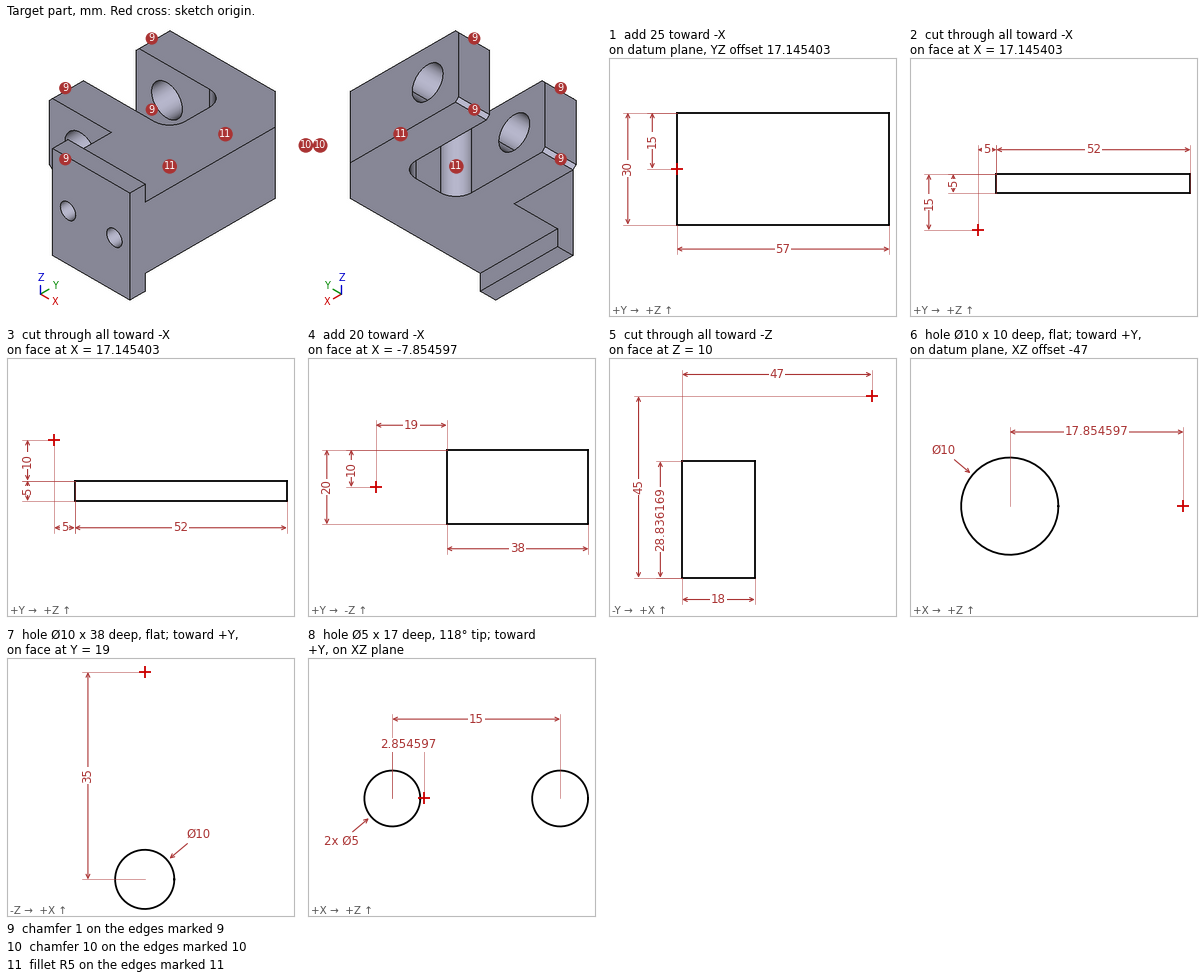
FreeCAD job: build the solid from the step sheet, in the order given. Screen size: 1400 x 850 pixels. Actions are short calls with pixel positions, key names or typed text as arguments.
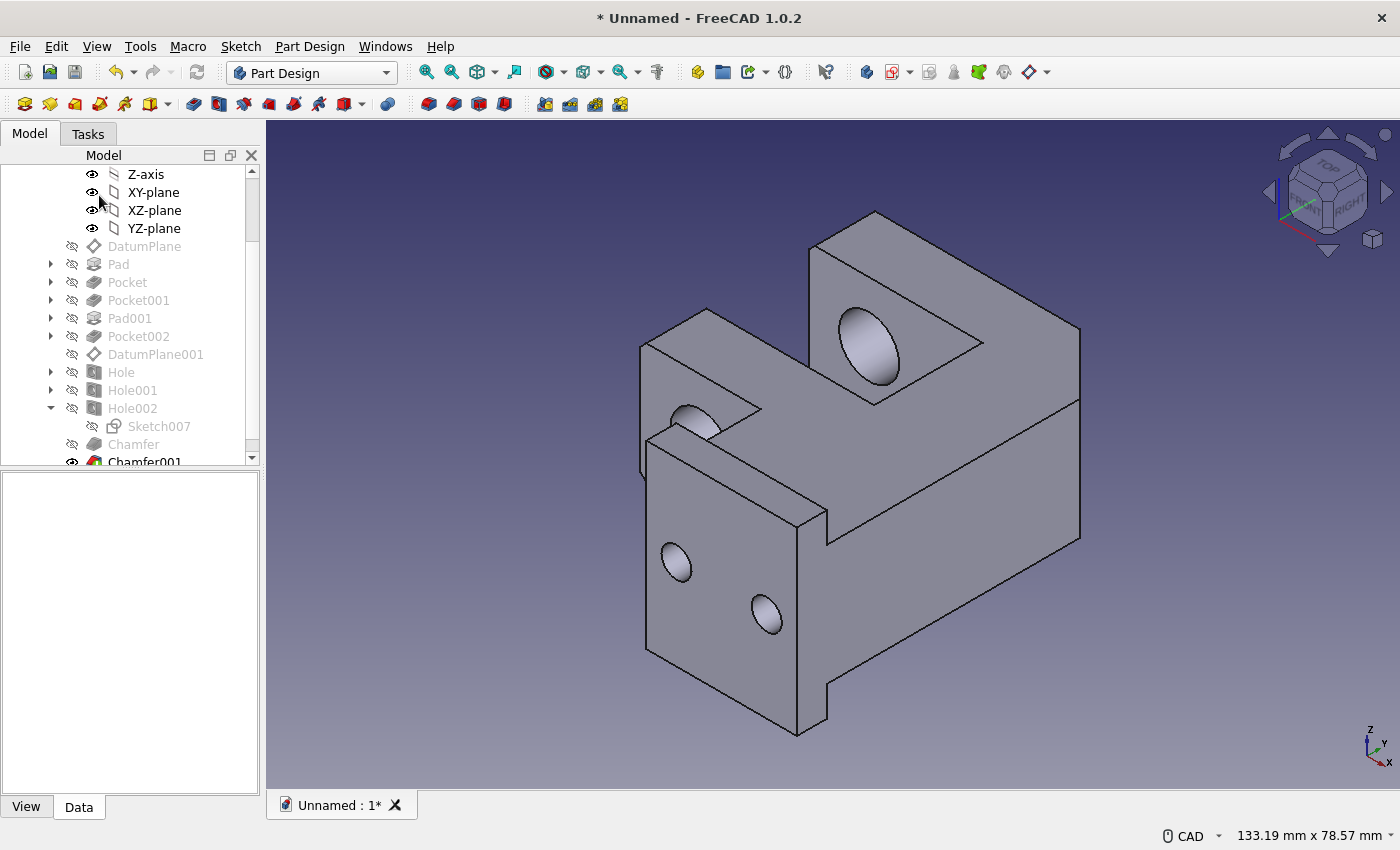
key(2)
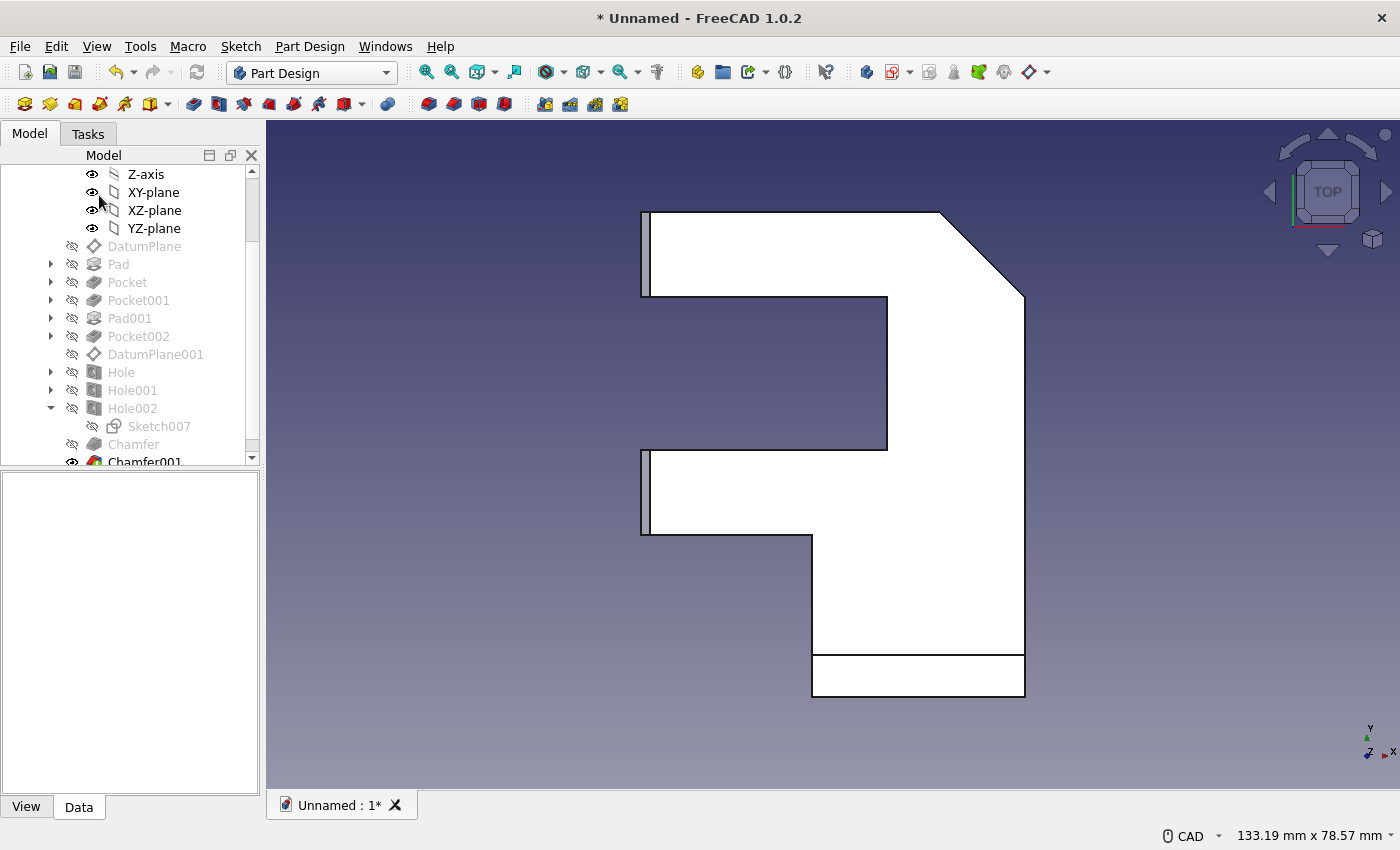
key(1)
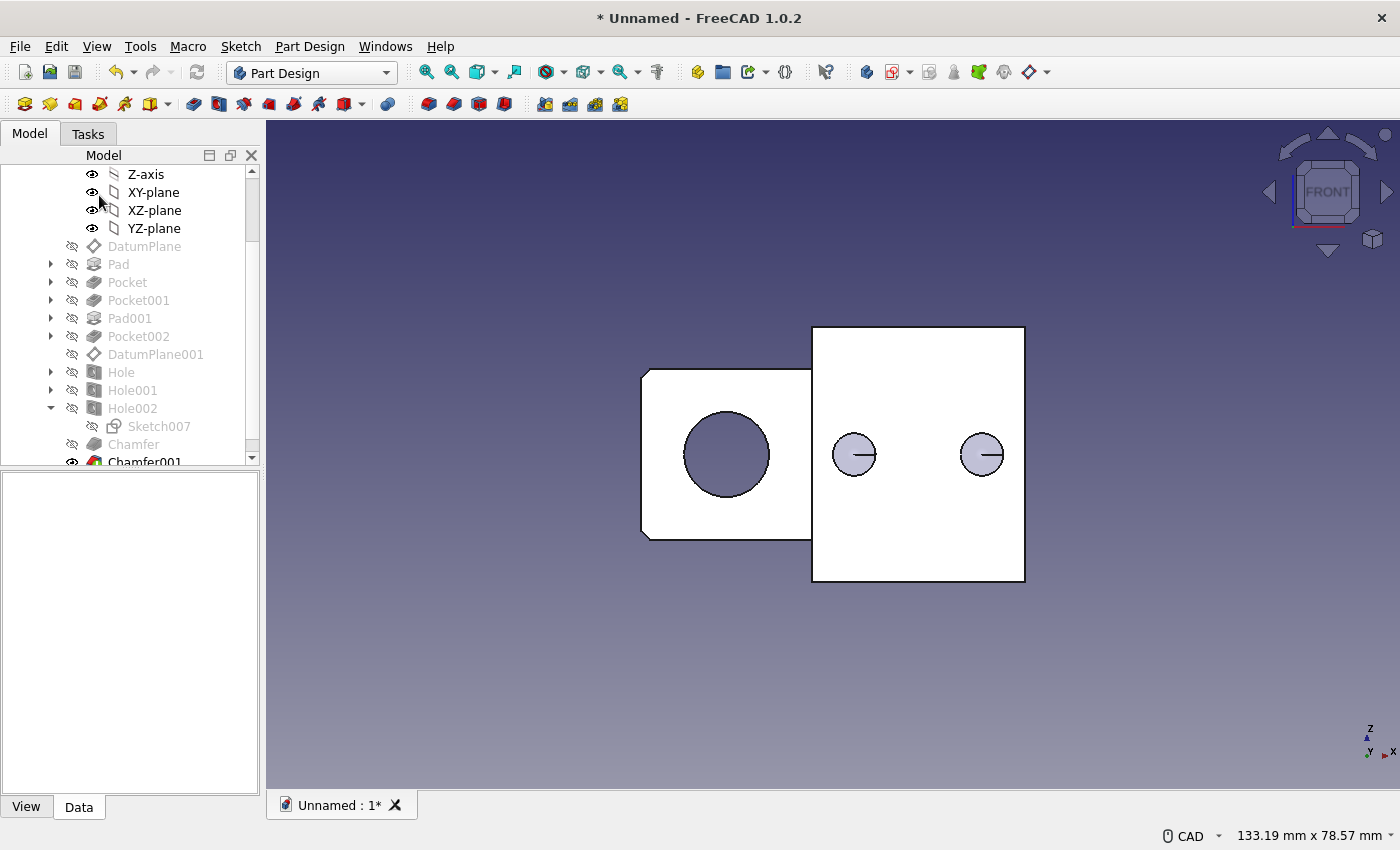
click(427, 72)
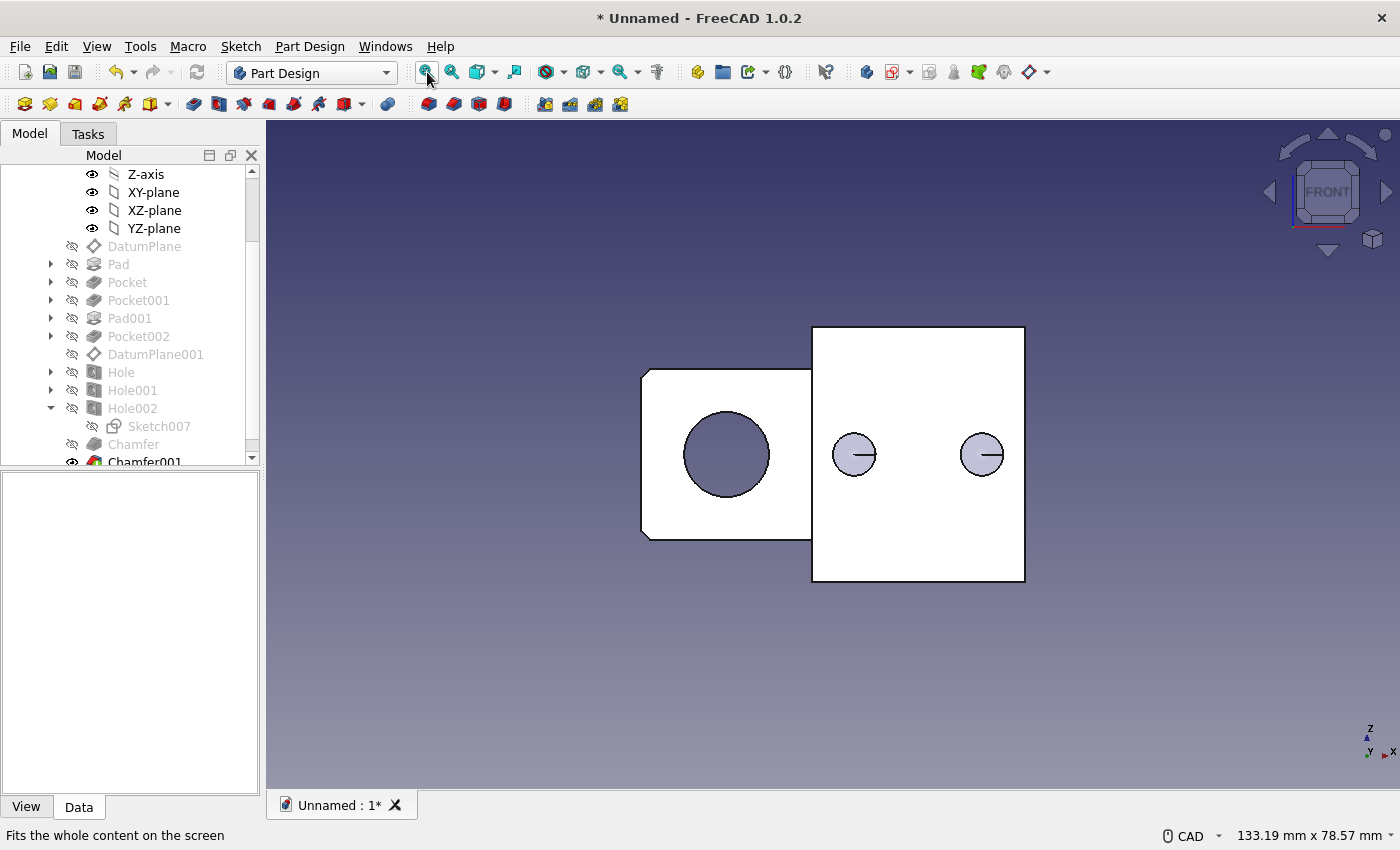
key(3)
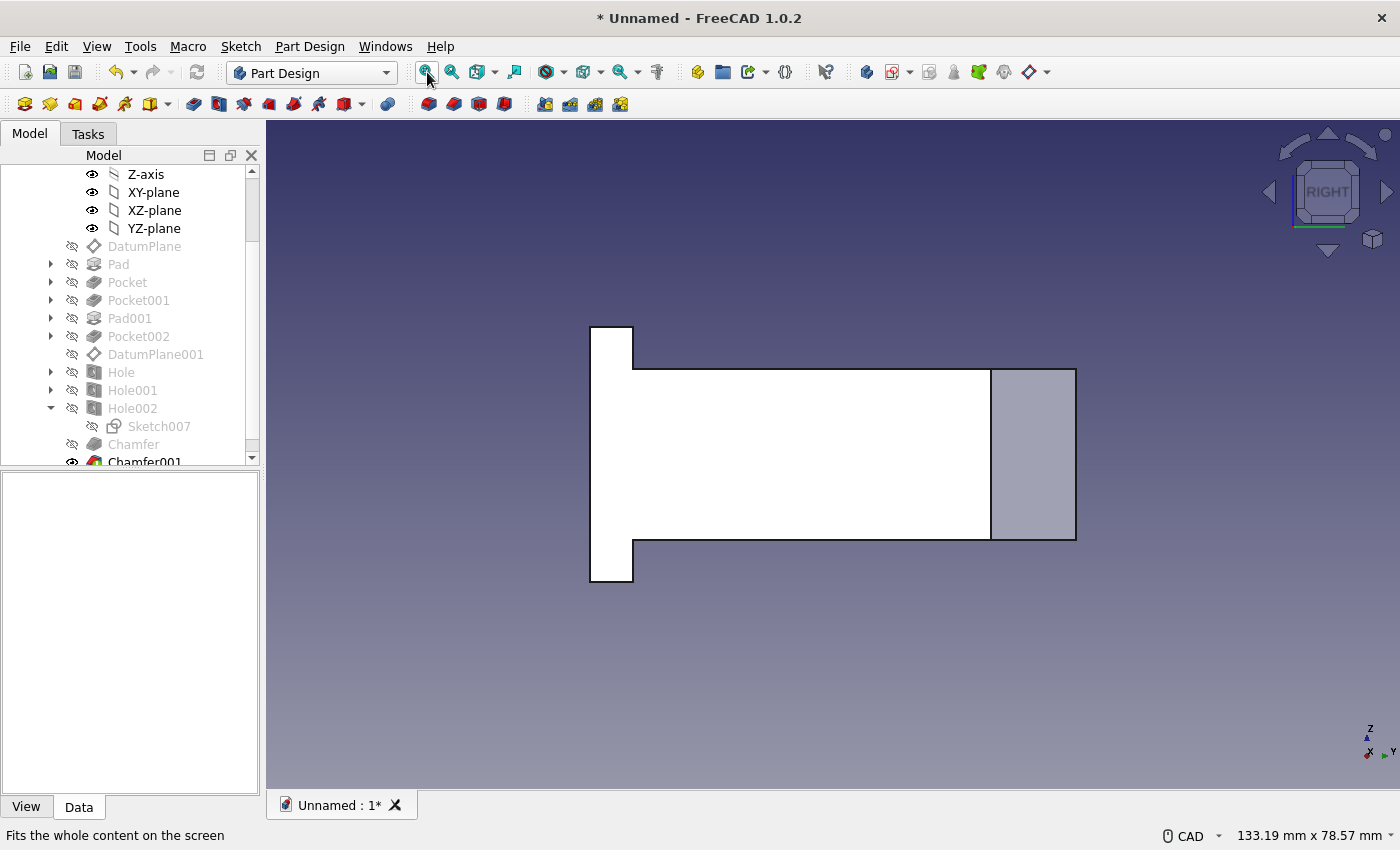
click(427, 72)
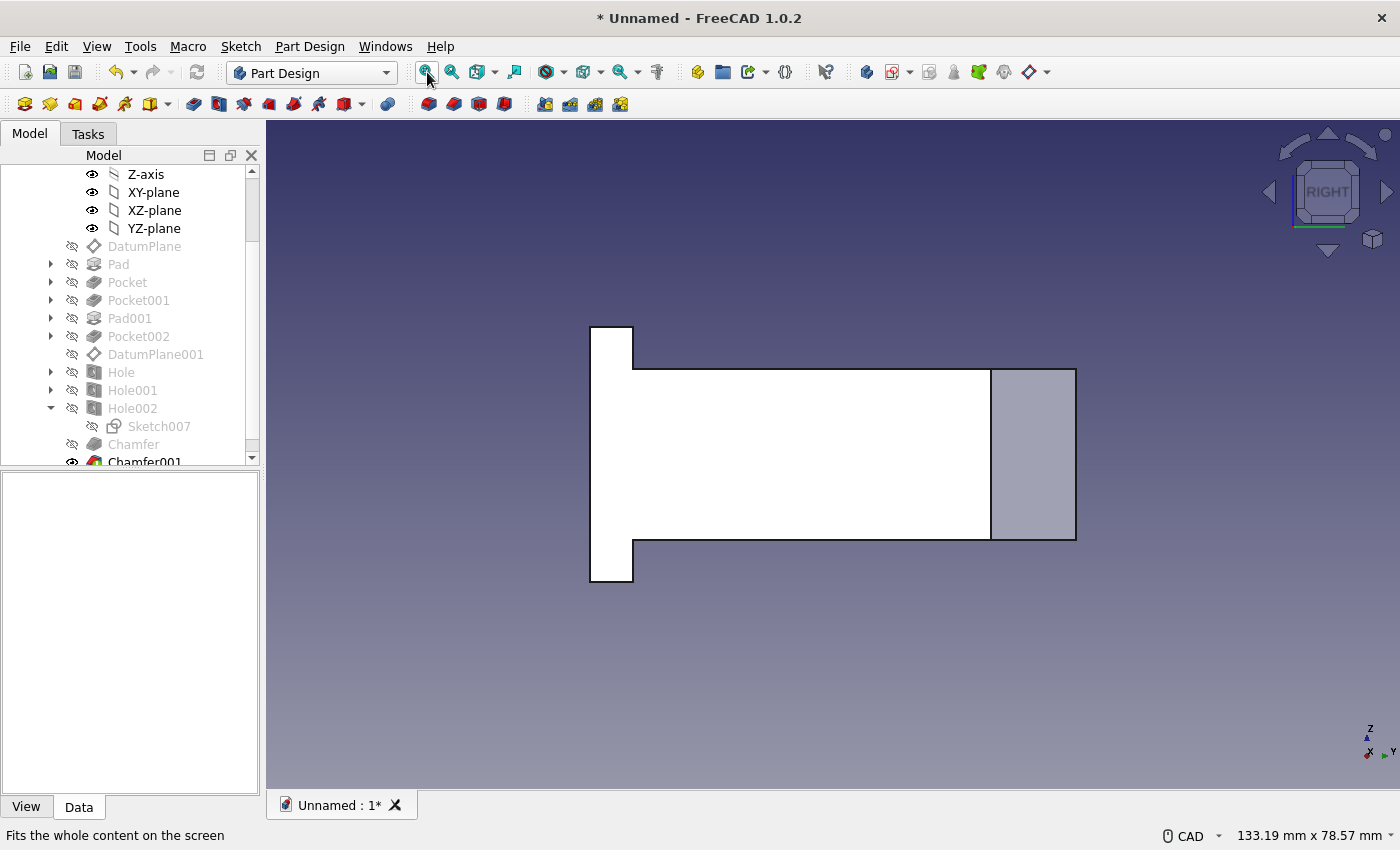
key(5)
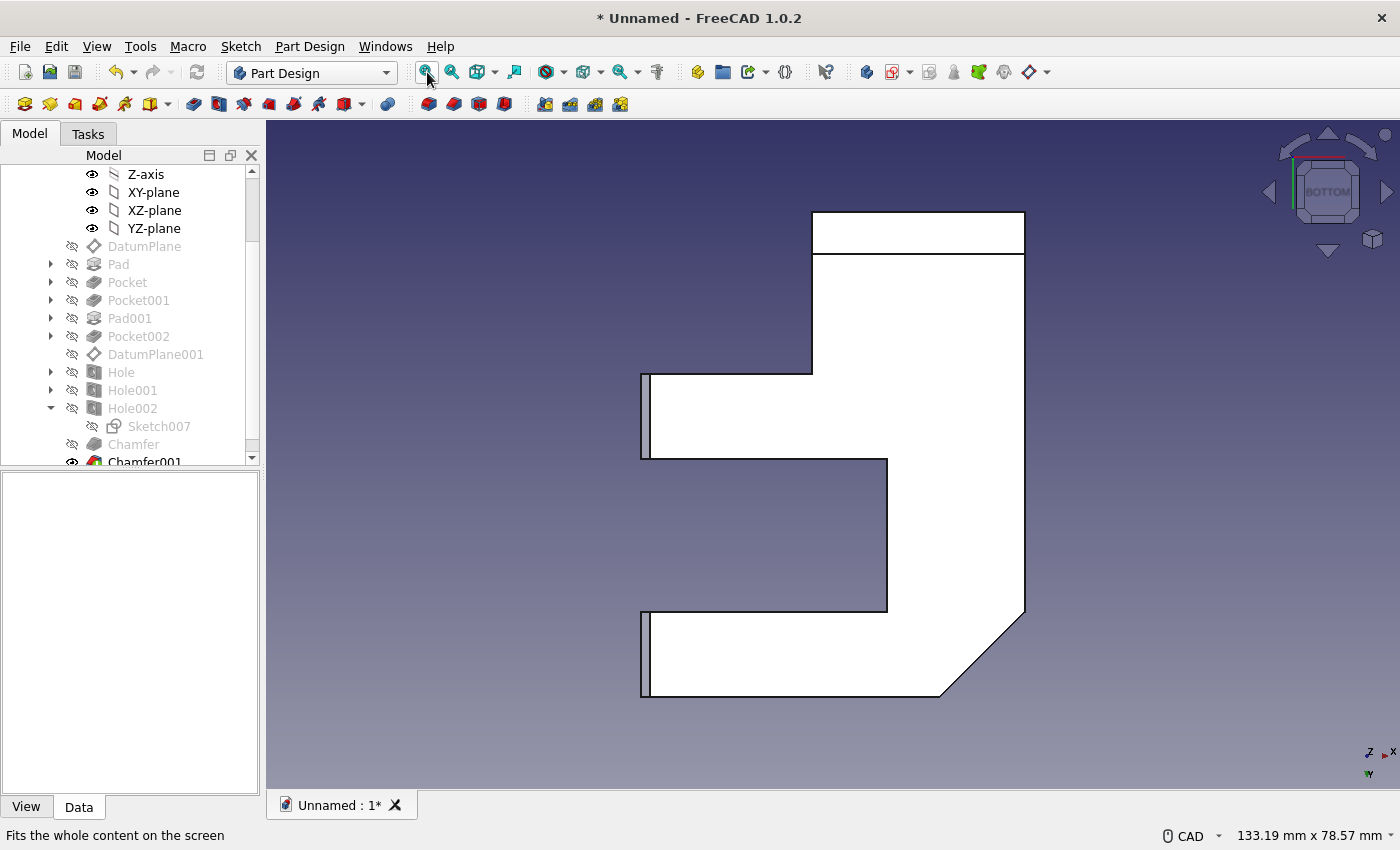
key(4)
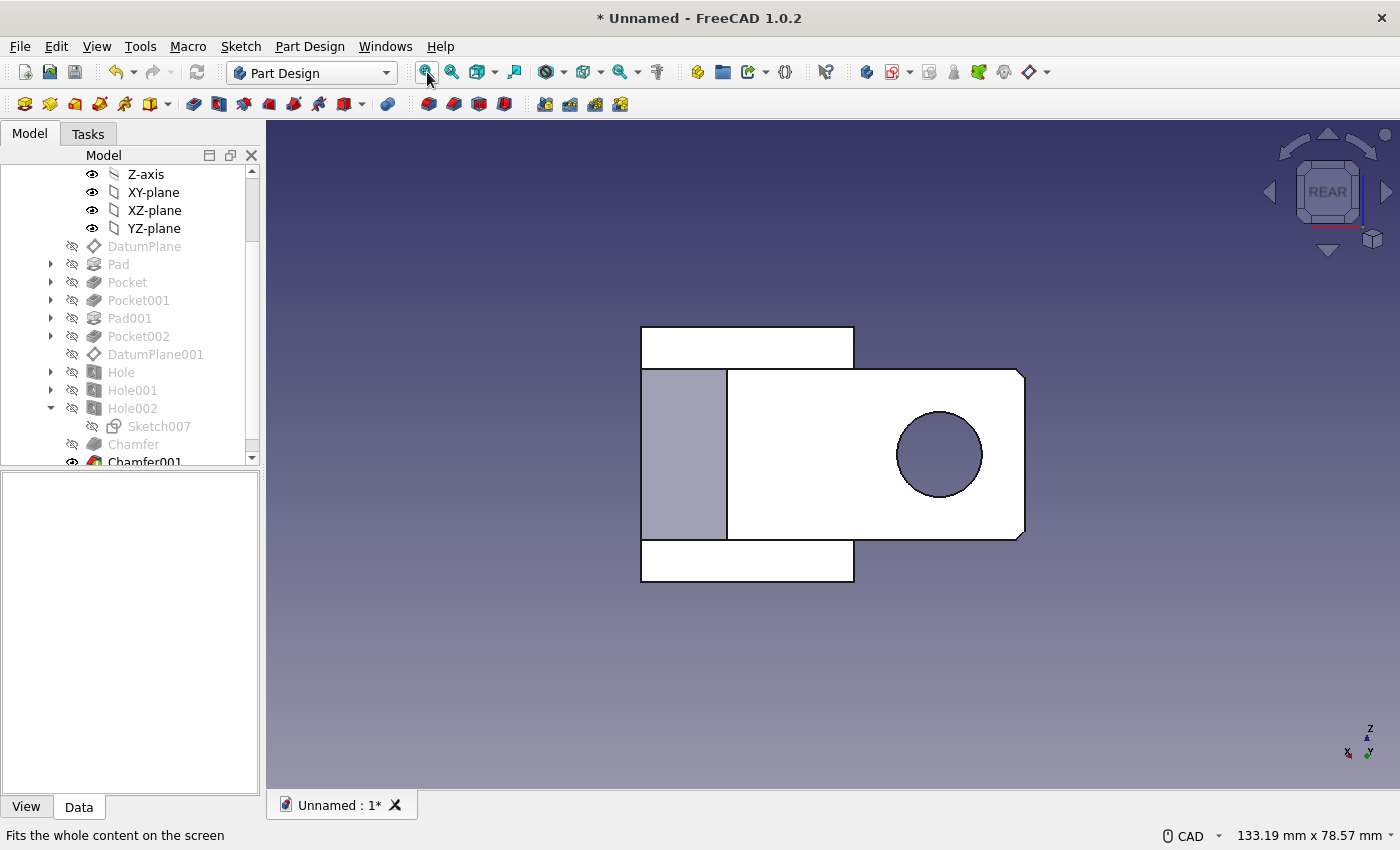
click(427, 72)